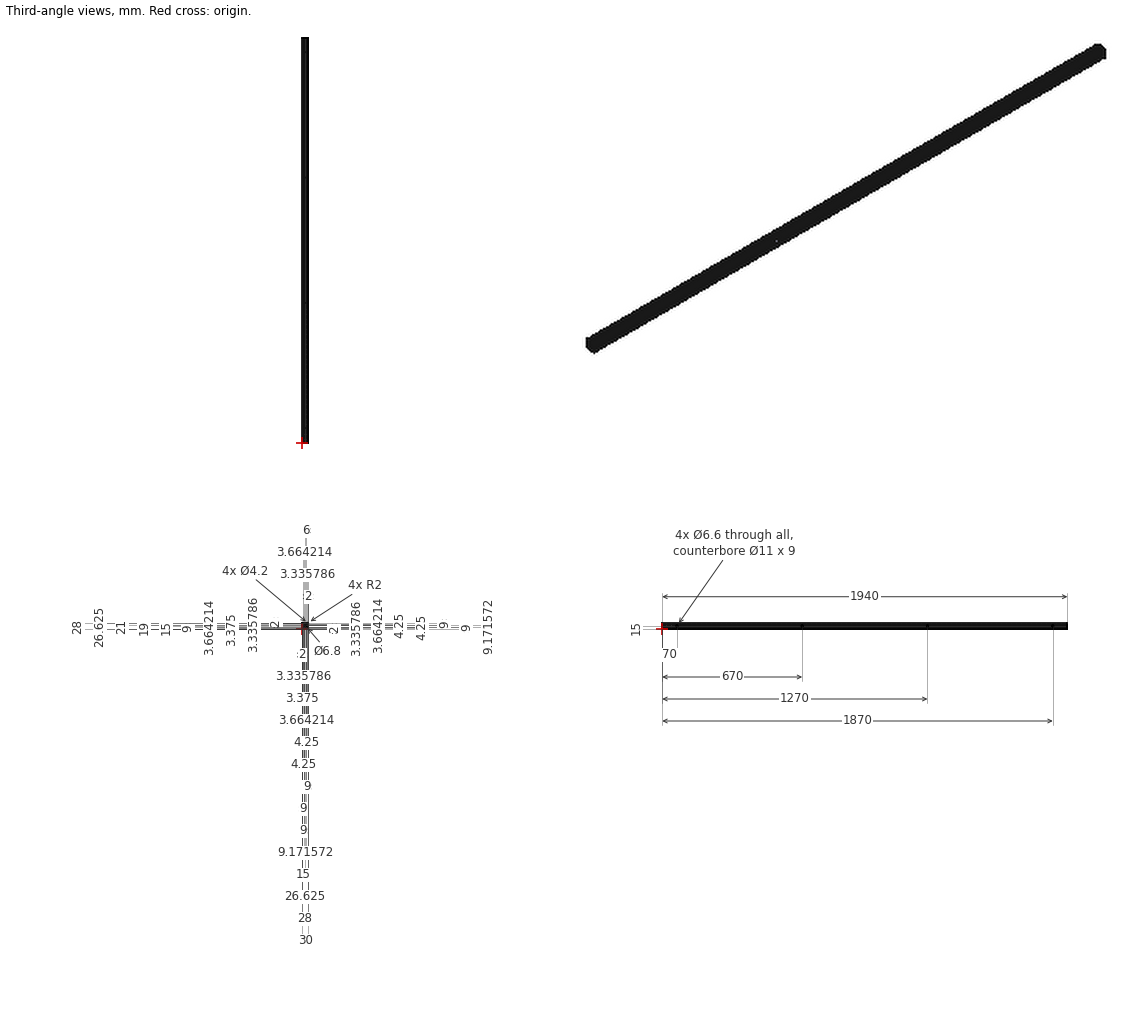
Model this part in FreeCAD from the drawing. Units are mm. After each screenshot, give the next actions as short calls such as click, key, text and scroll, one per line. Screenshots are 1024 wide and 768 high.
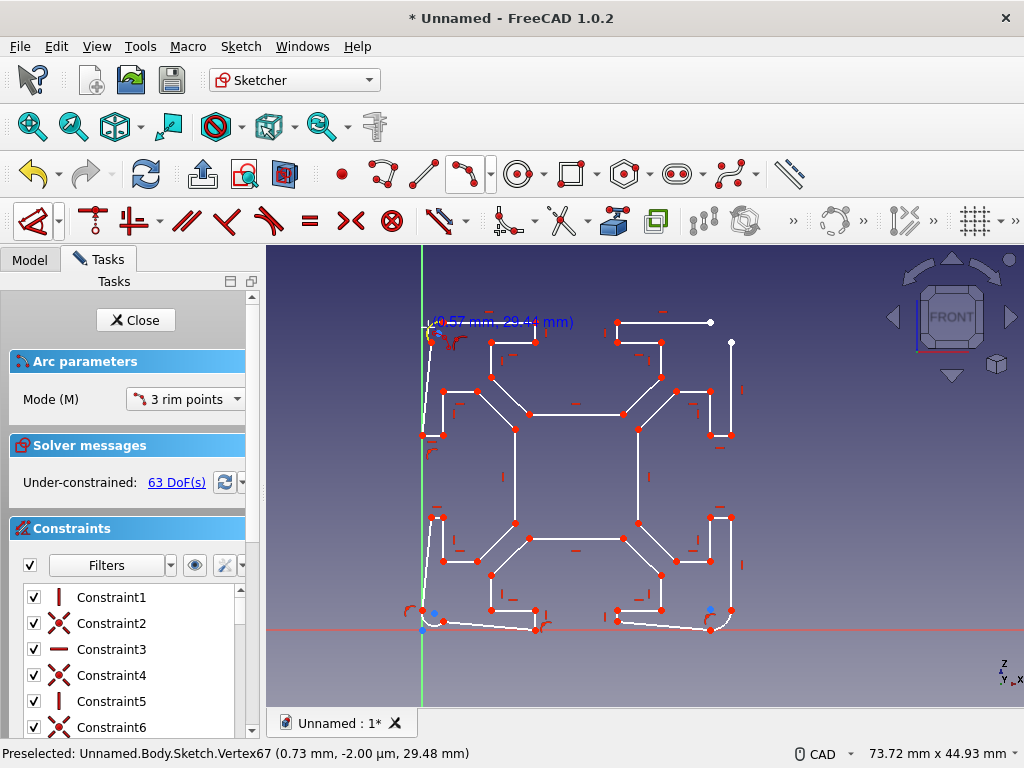
click(710, 323)
click(731, 343)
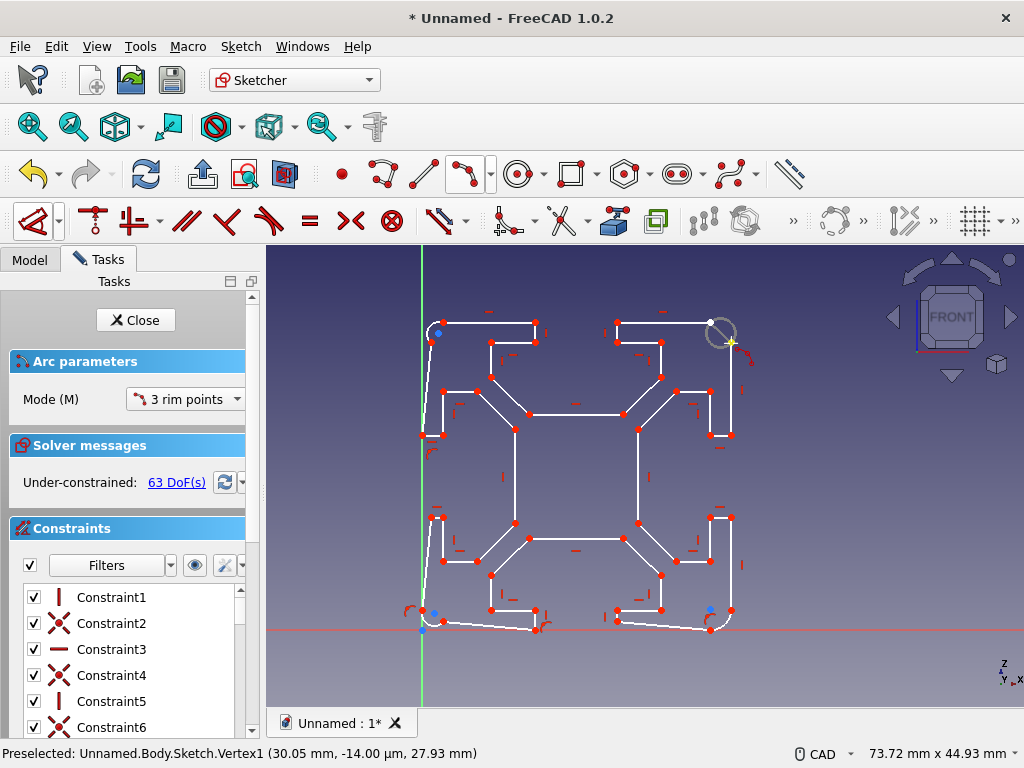
scroll(725, 328, up, 5)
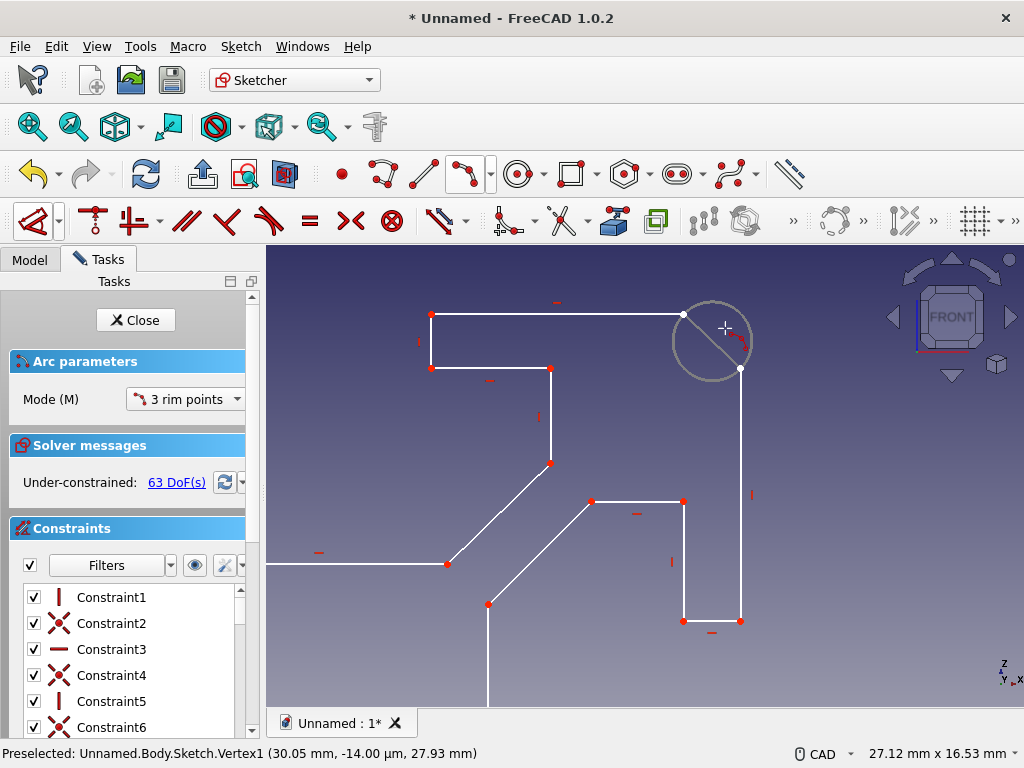
click(723, 327)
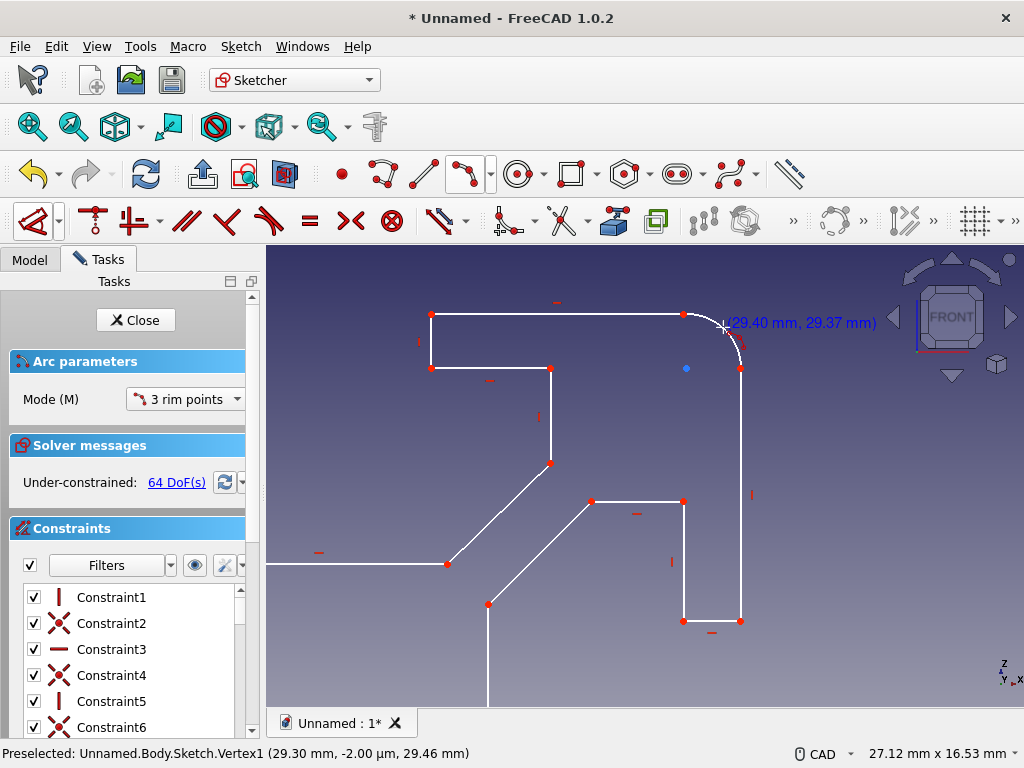
click(518, 174)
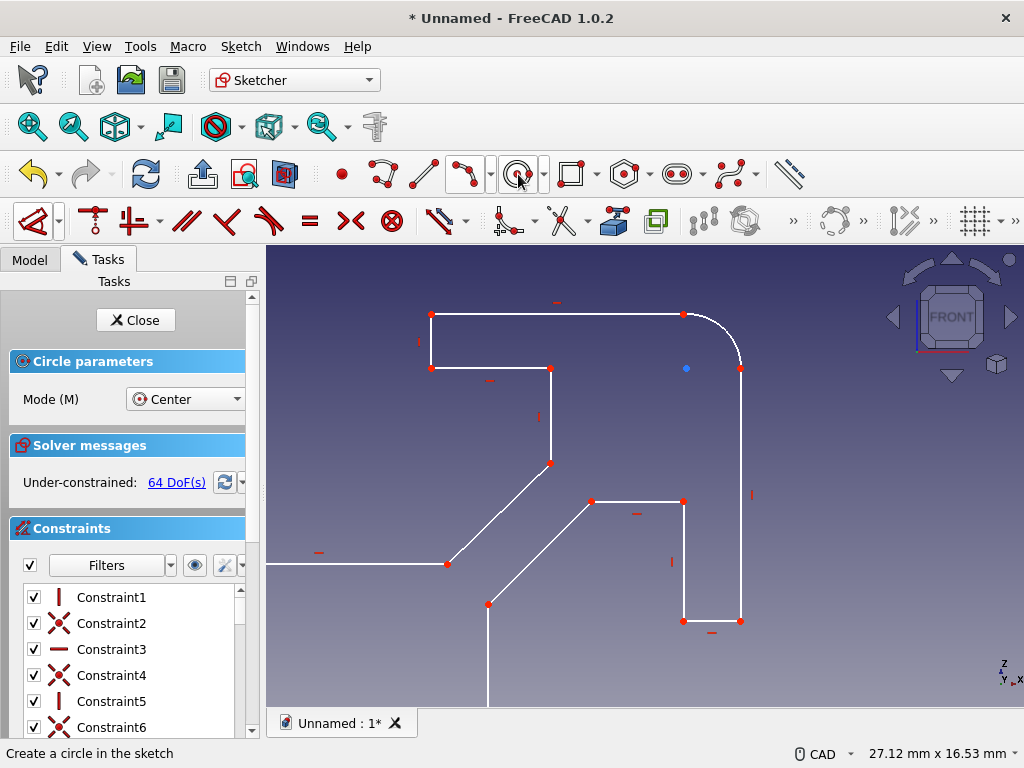
click(645, 405)
click(604, 363)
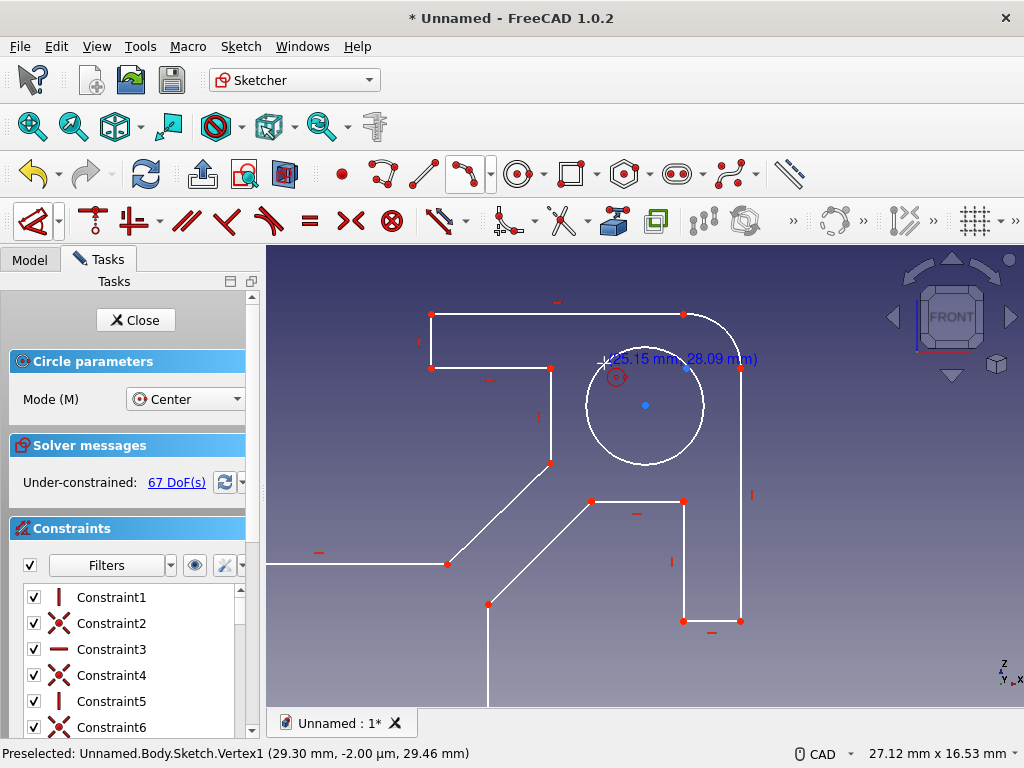
scroll(726, 328, down, 5)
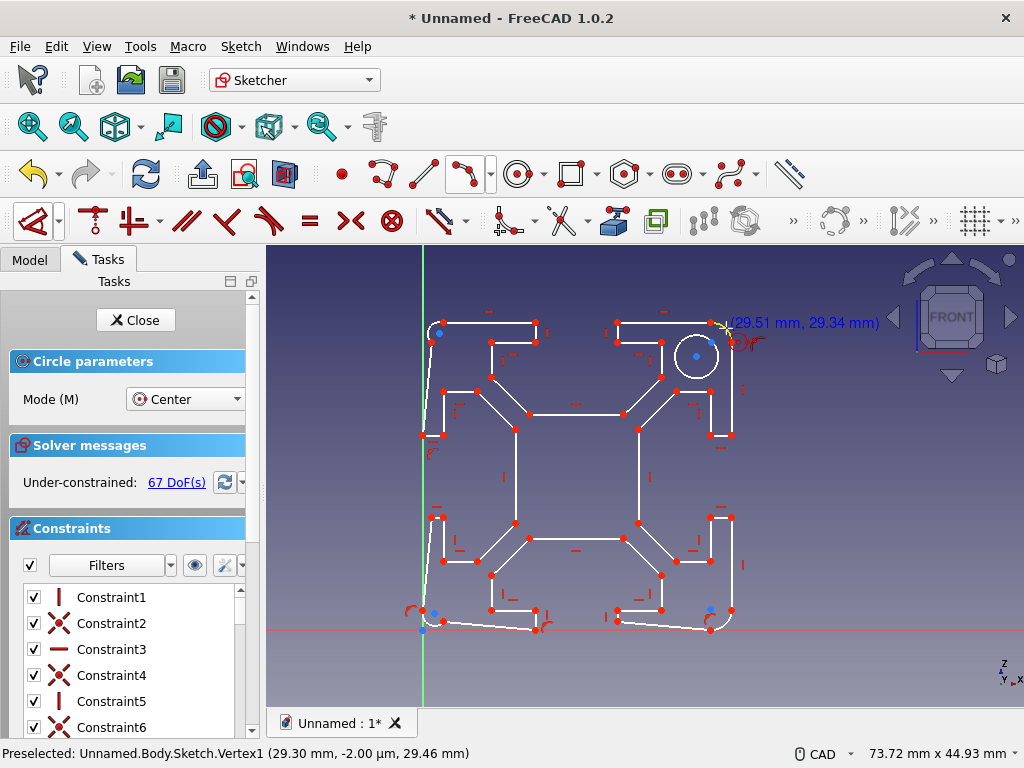
click(458, 356)
click(473, 341)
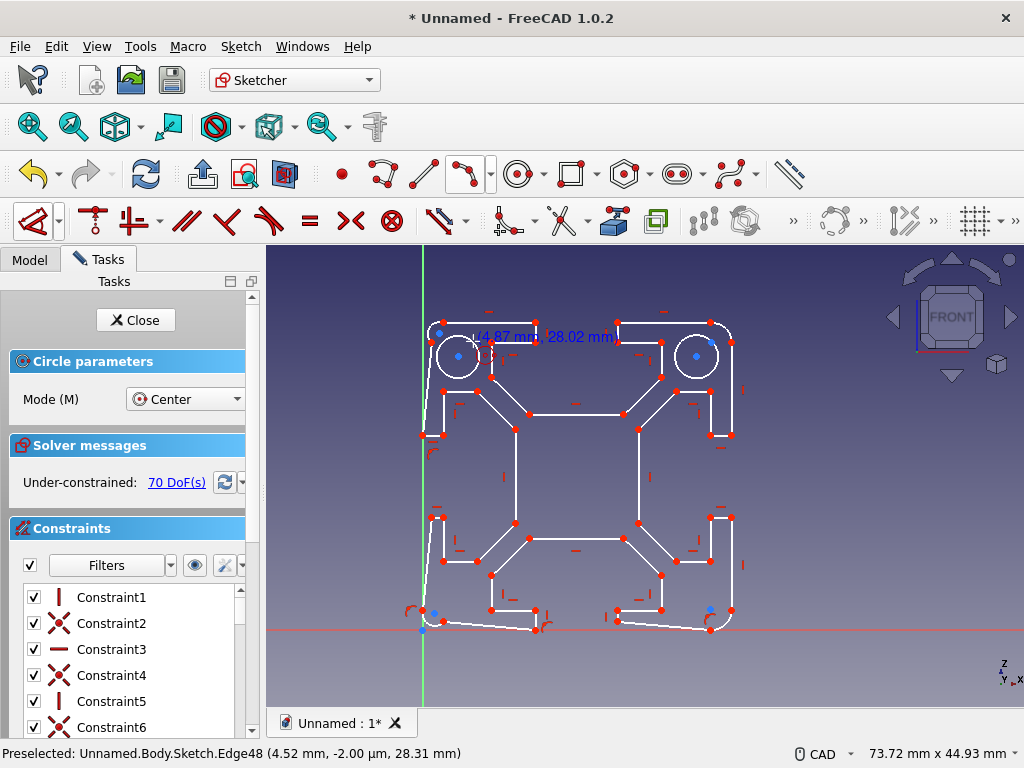
click(697, 595)
click(712, 580)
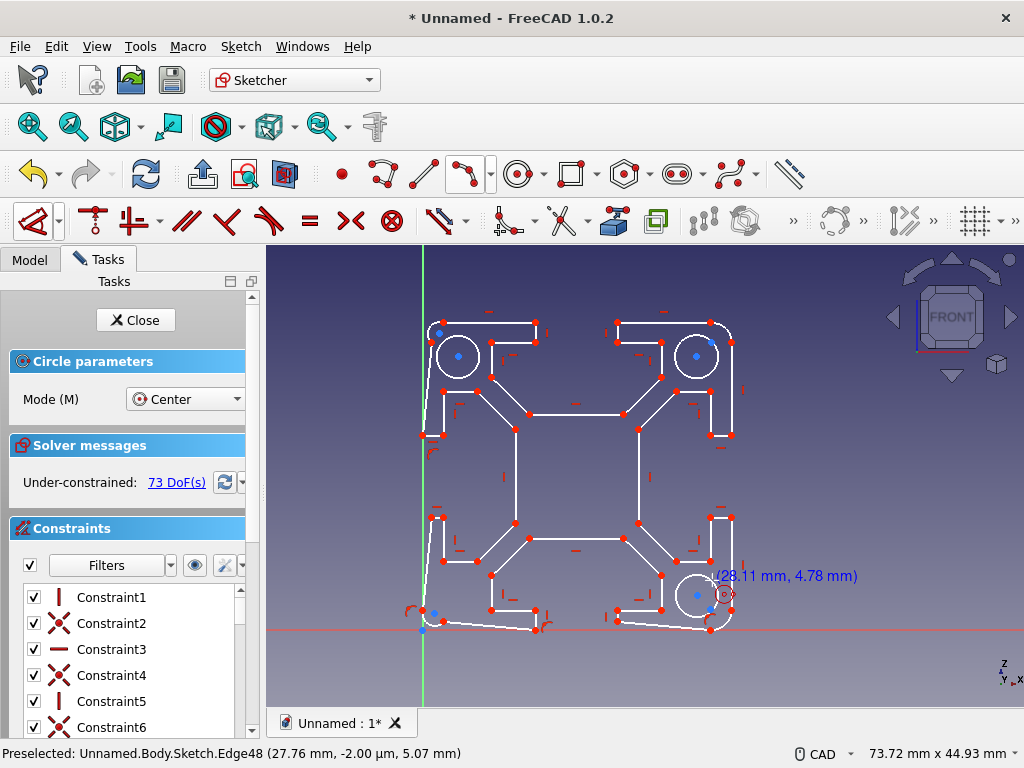
click(577, 476)
click(602, 451)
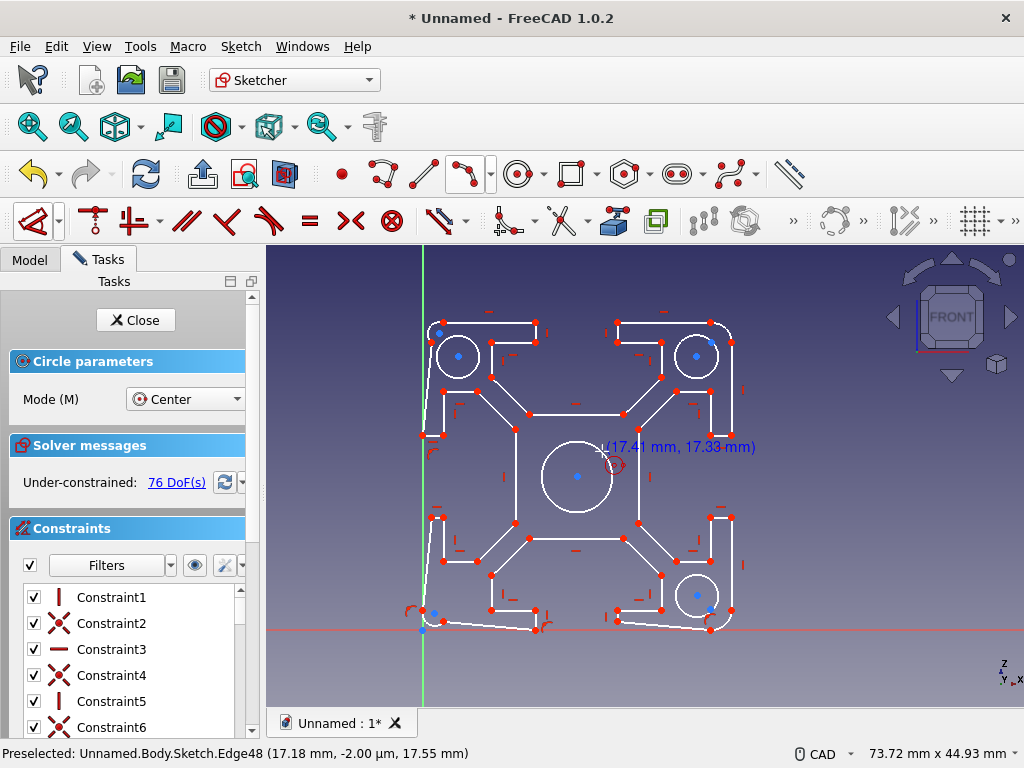
click(458, 595)
click(473, 580)
key(Escape)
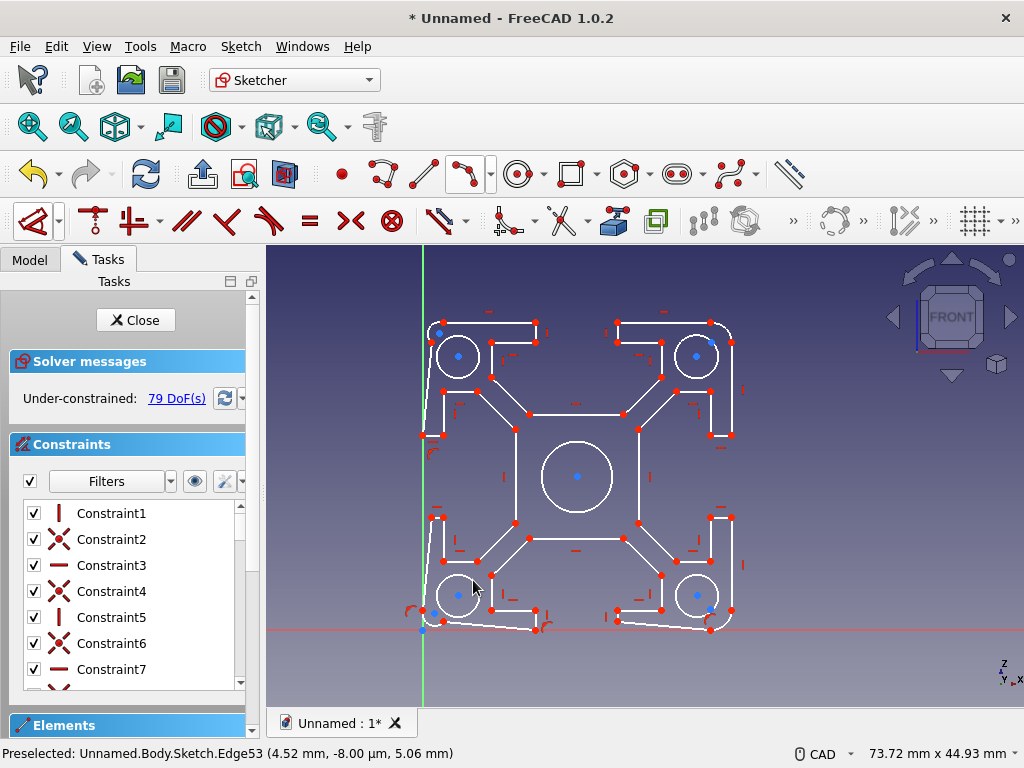
click(732, 371)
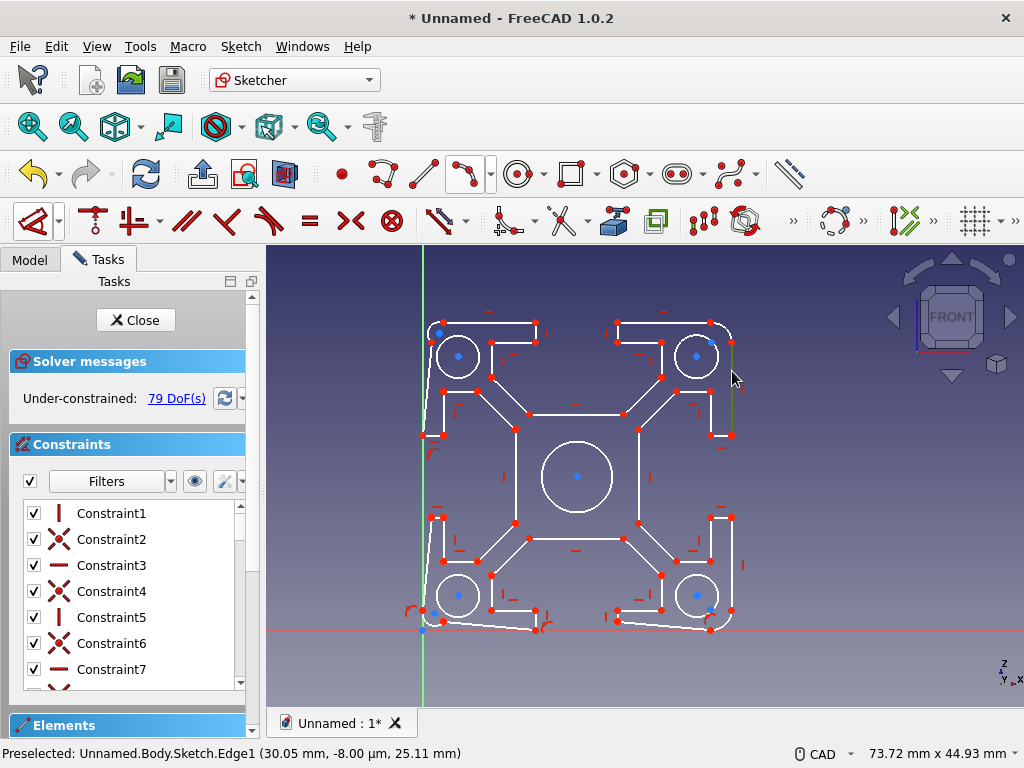
scroll(730, 334, up, 2)